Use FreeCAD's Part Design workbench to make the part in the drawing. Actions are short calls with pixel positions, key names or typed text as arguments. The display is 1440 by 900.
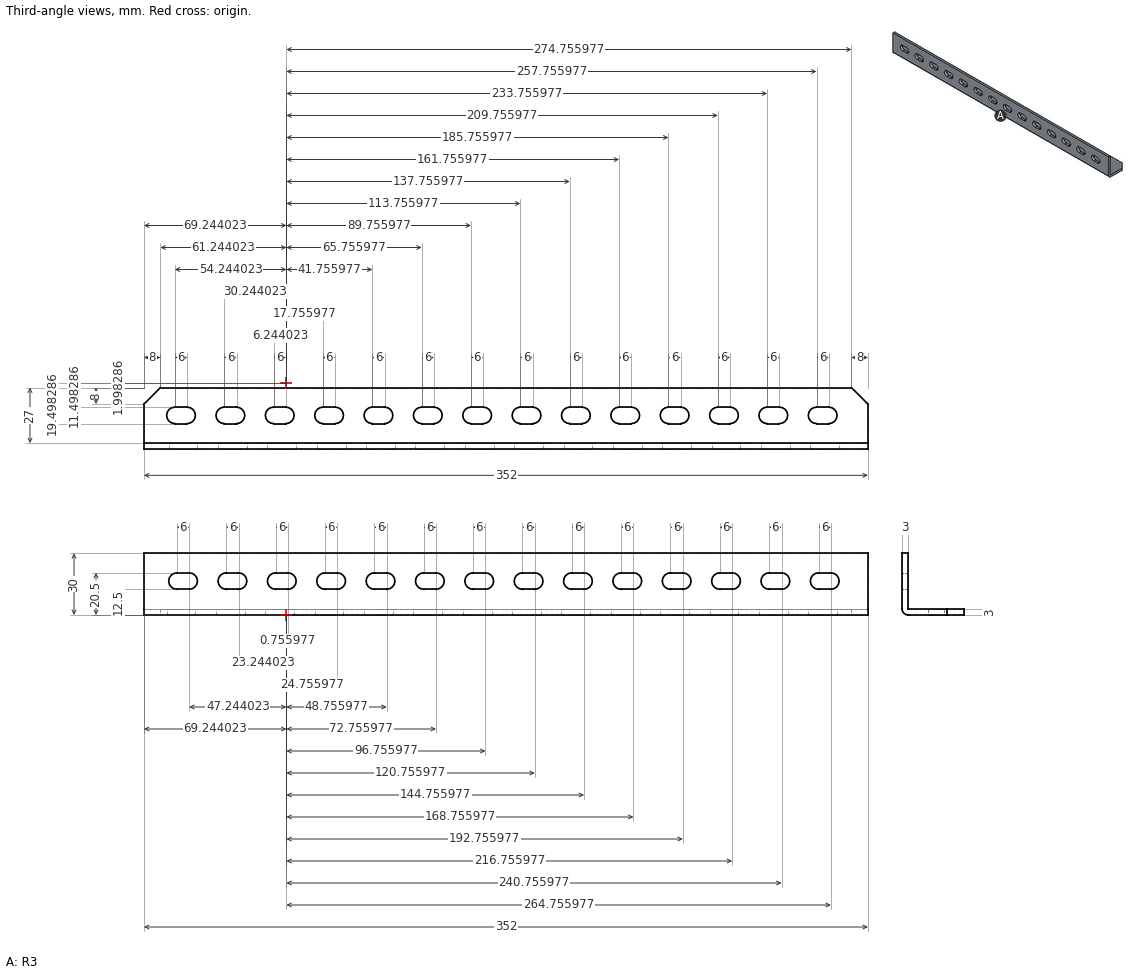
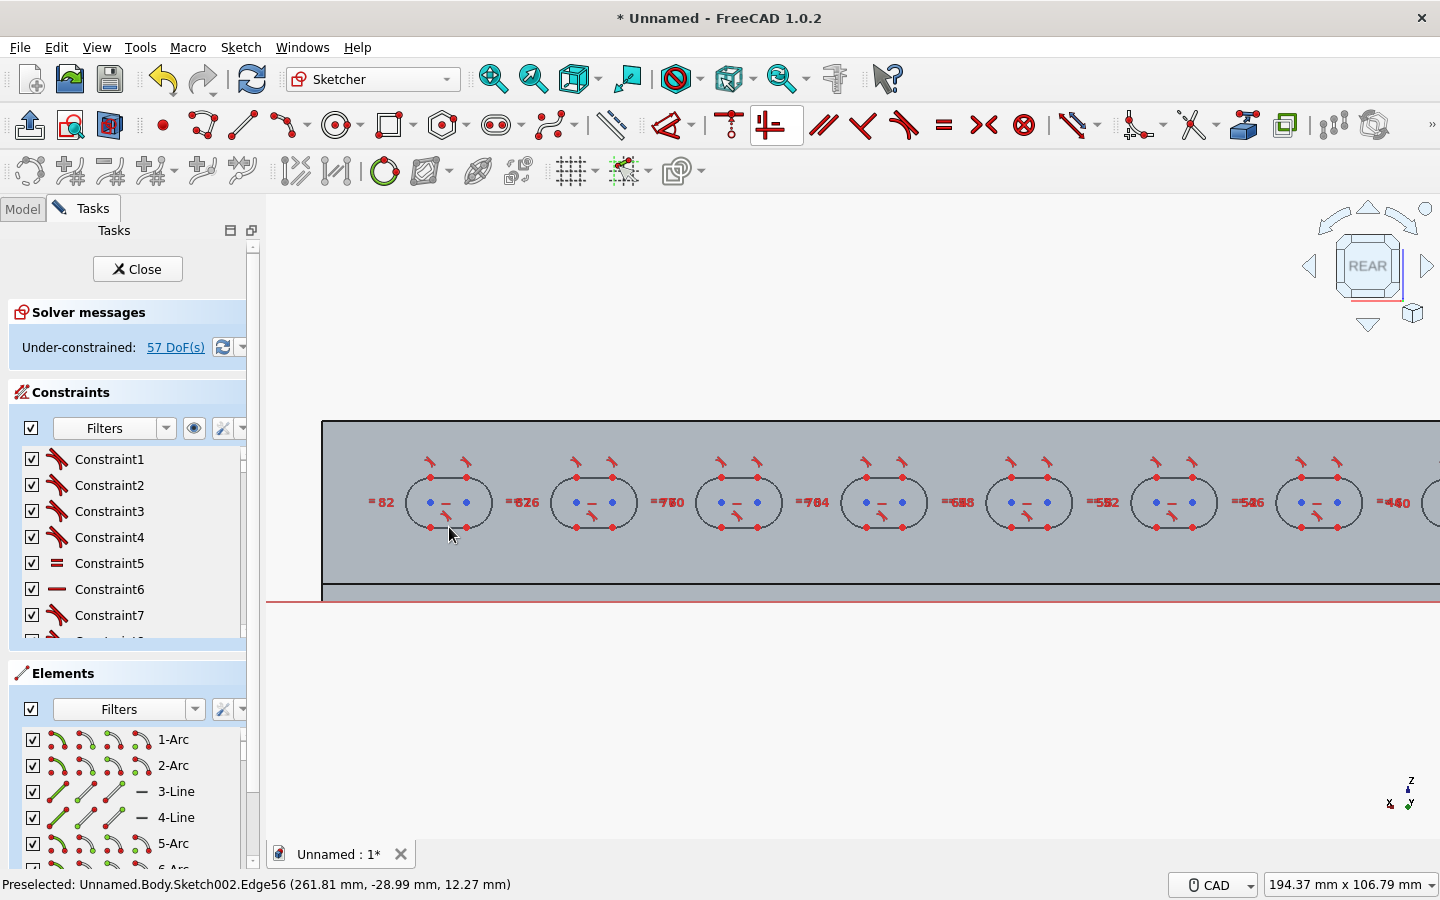
scroll(431, 503, down, 5)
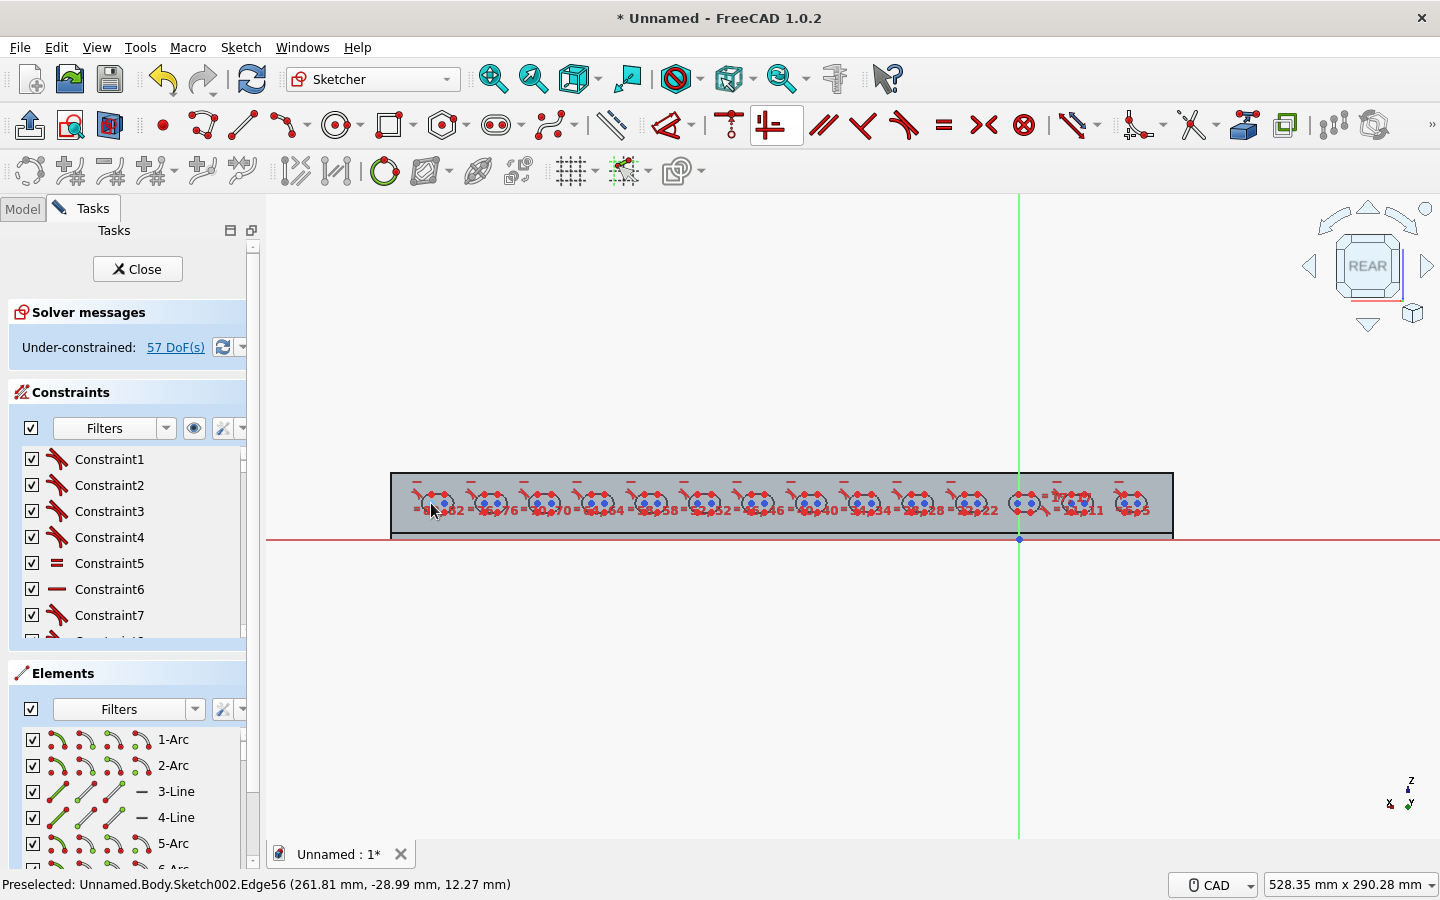
scroll(1027, 495, up, 7)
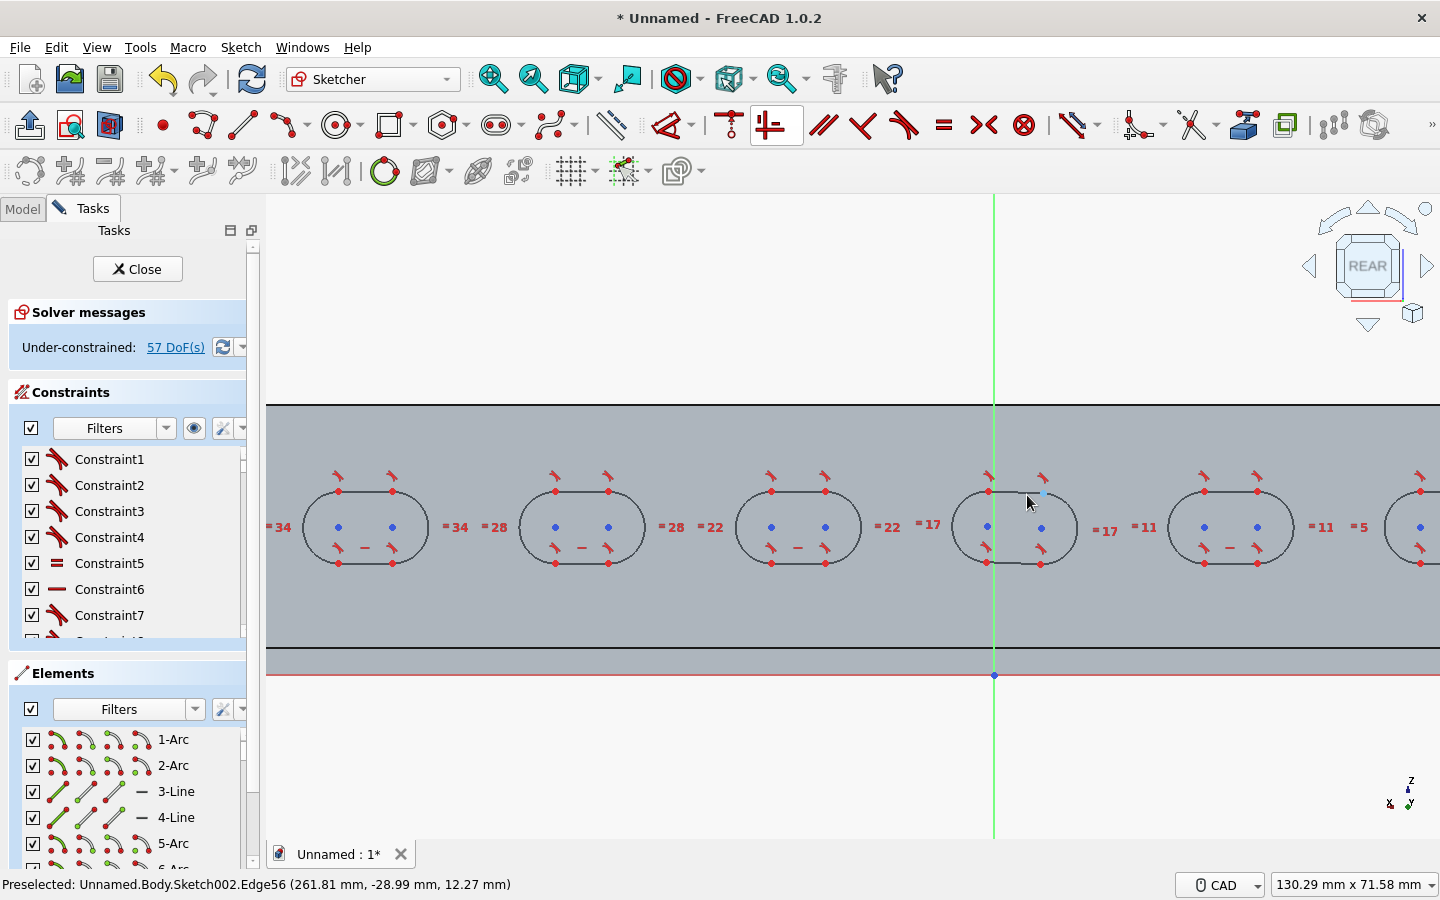
click(1027, 493)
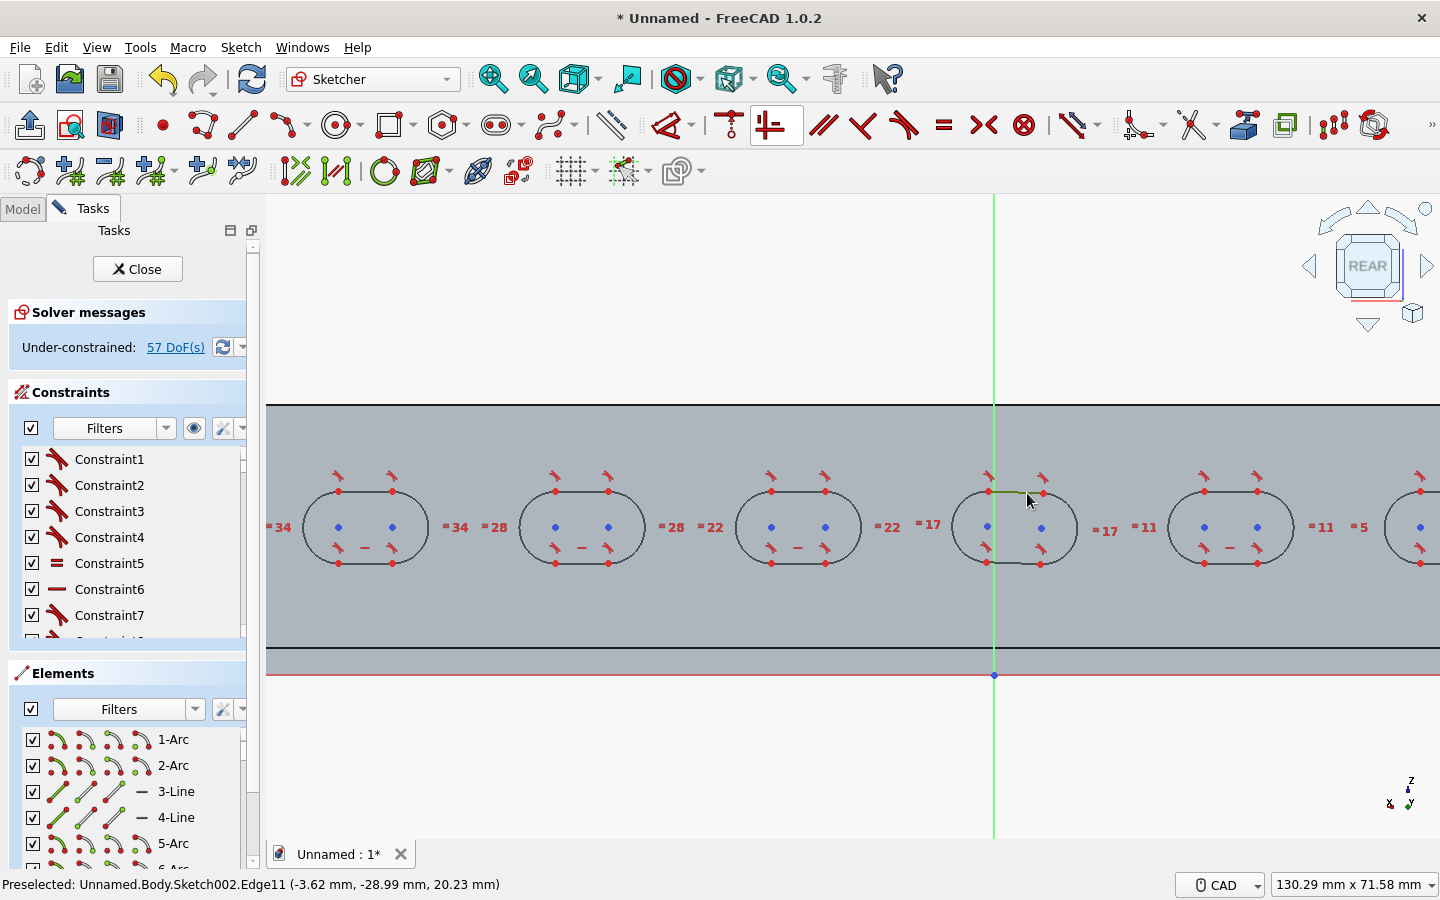
click(798, 126)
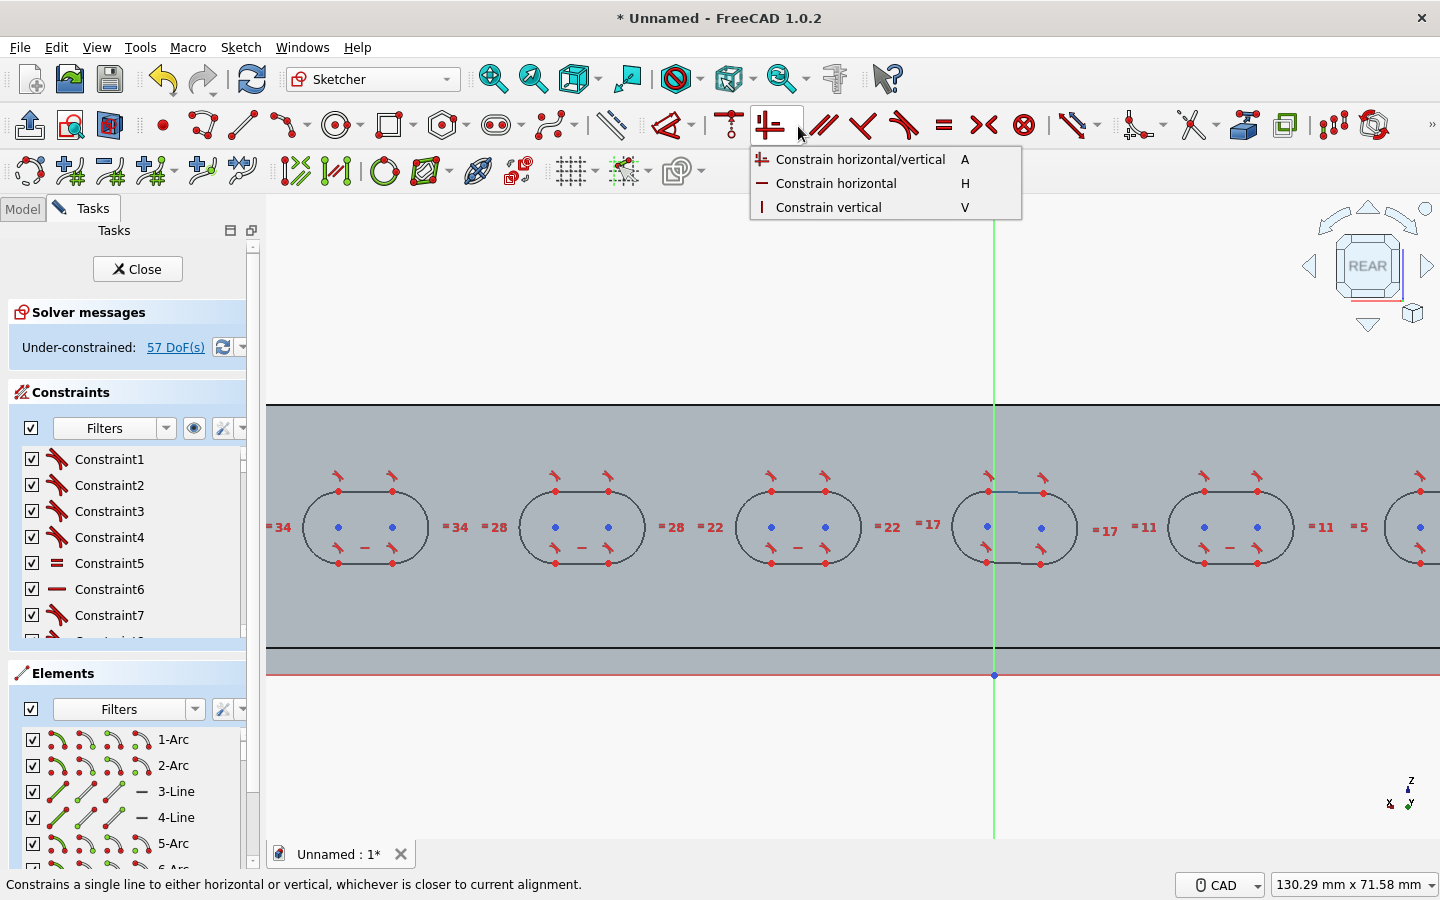
click(886, 183)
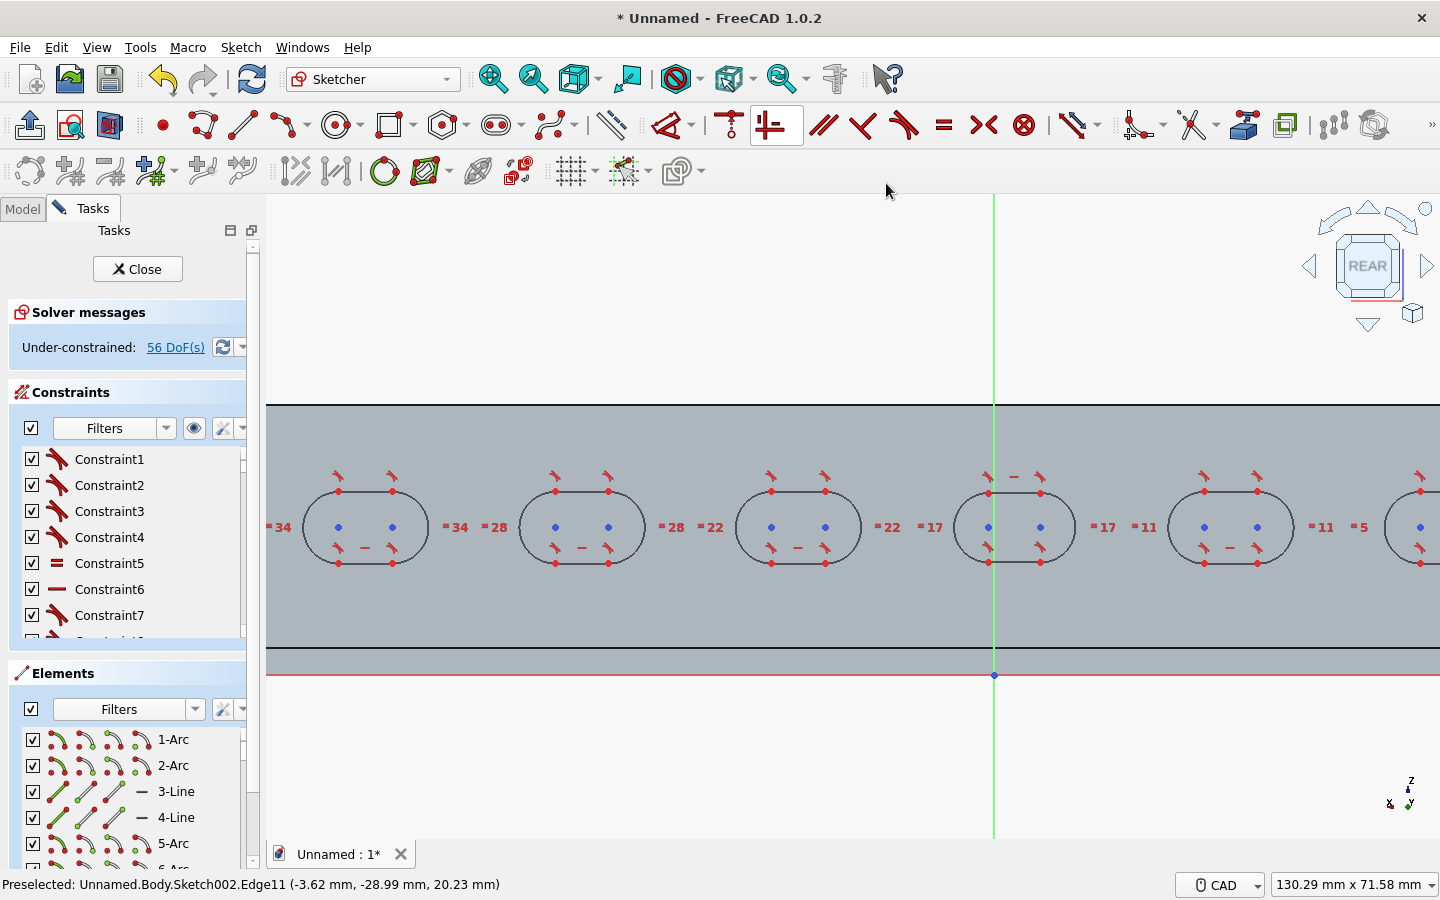
scroll(1028, 495, down, 7)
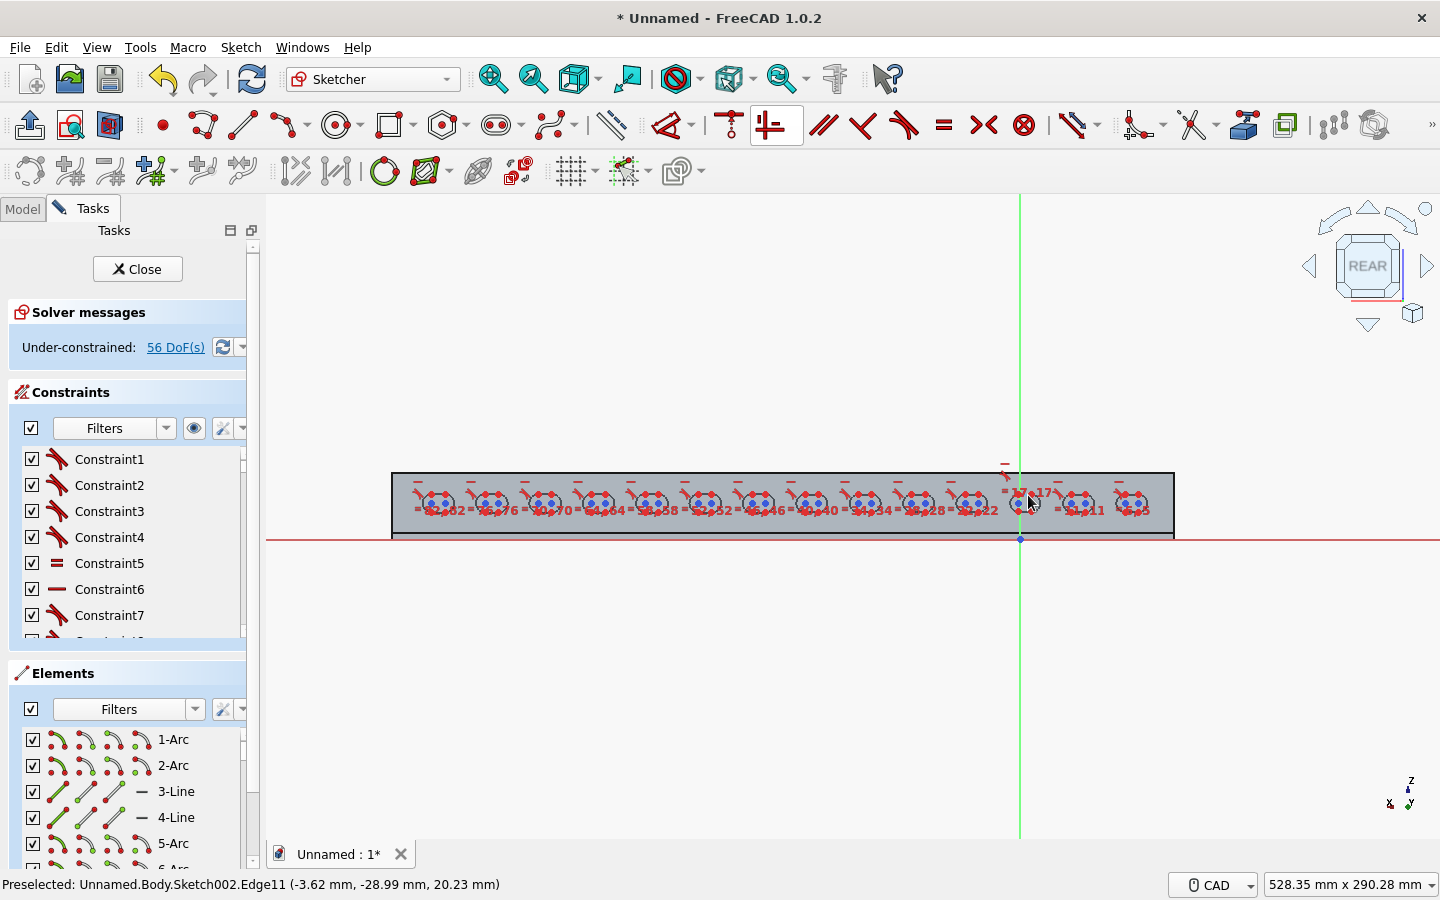
scroll(1118, 498, up, 3)